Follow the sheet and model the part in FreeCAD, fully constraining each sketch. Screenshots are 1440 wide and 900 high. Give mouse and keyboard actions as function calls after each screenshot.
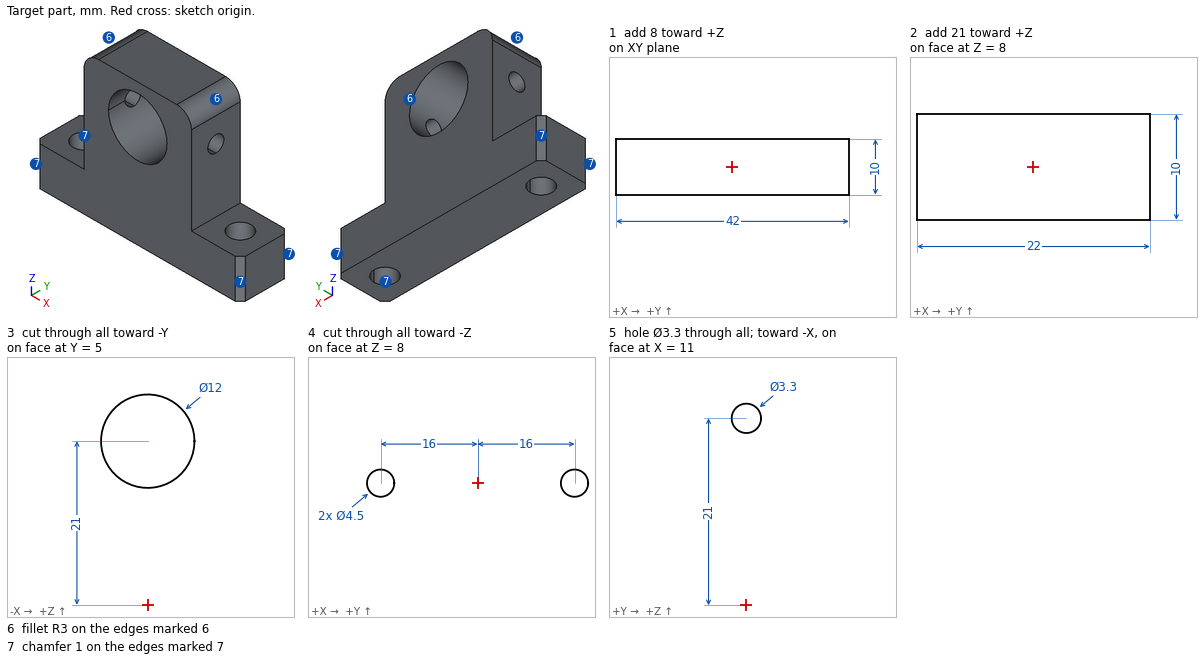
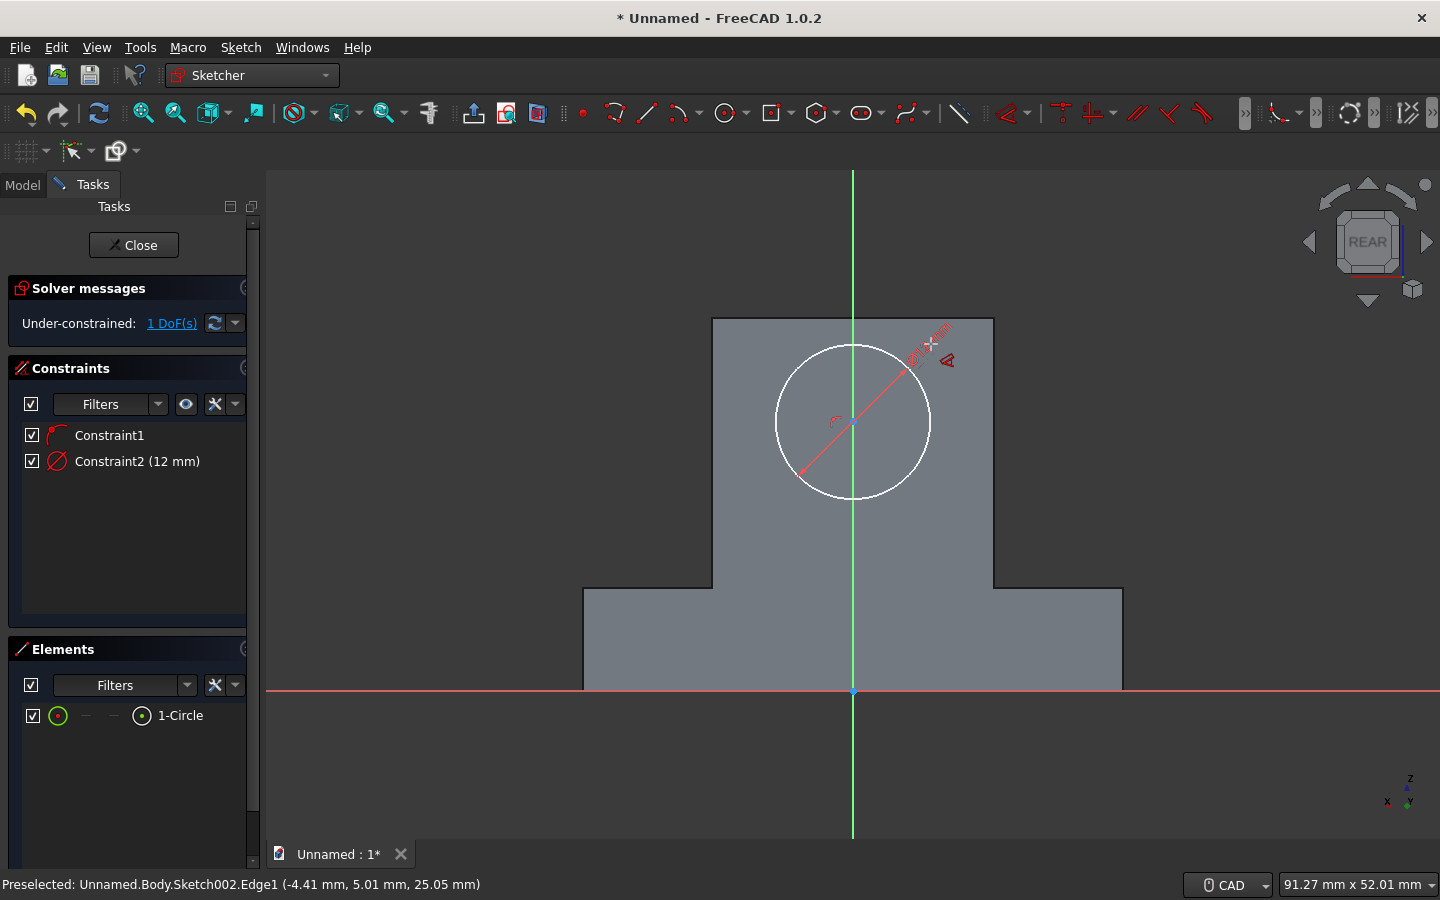
click(853, 422)
click(887, 557)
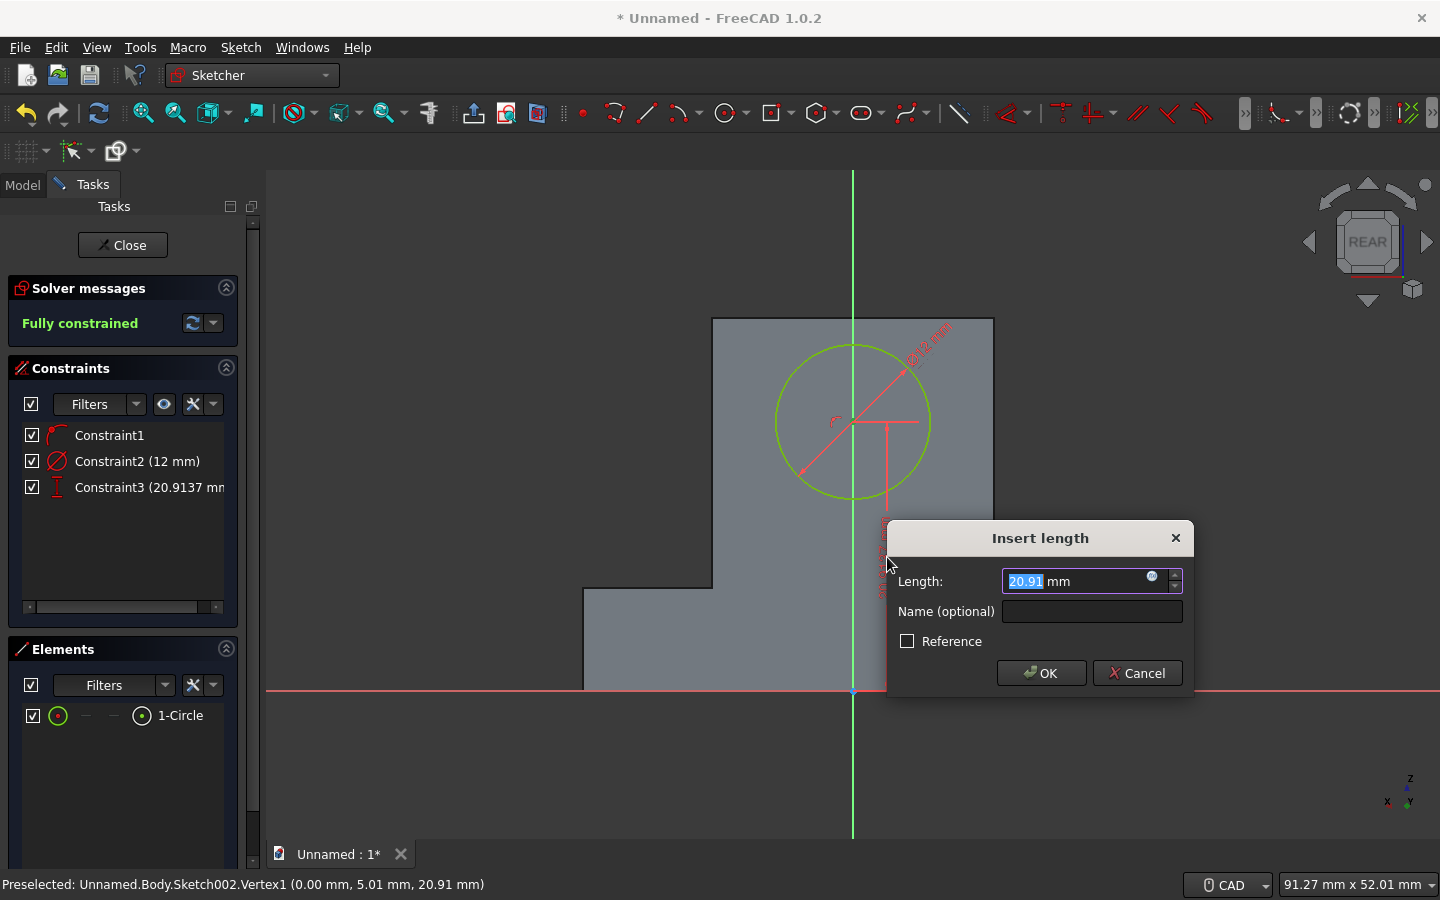
text(21)
key(Return)
key(Escape)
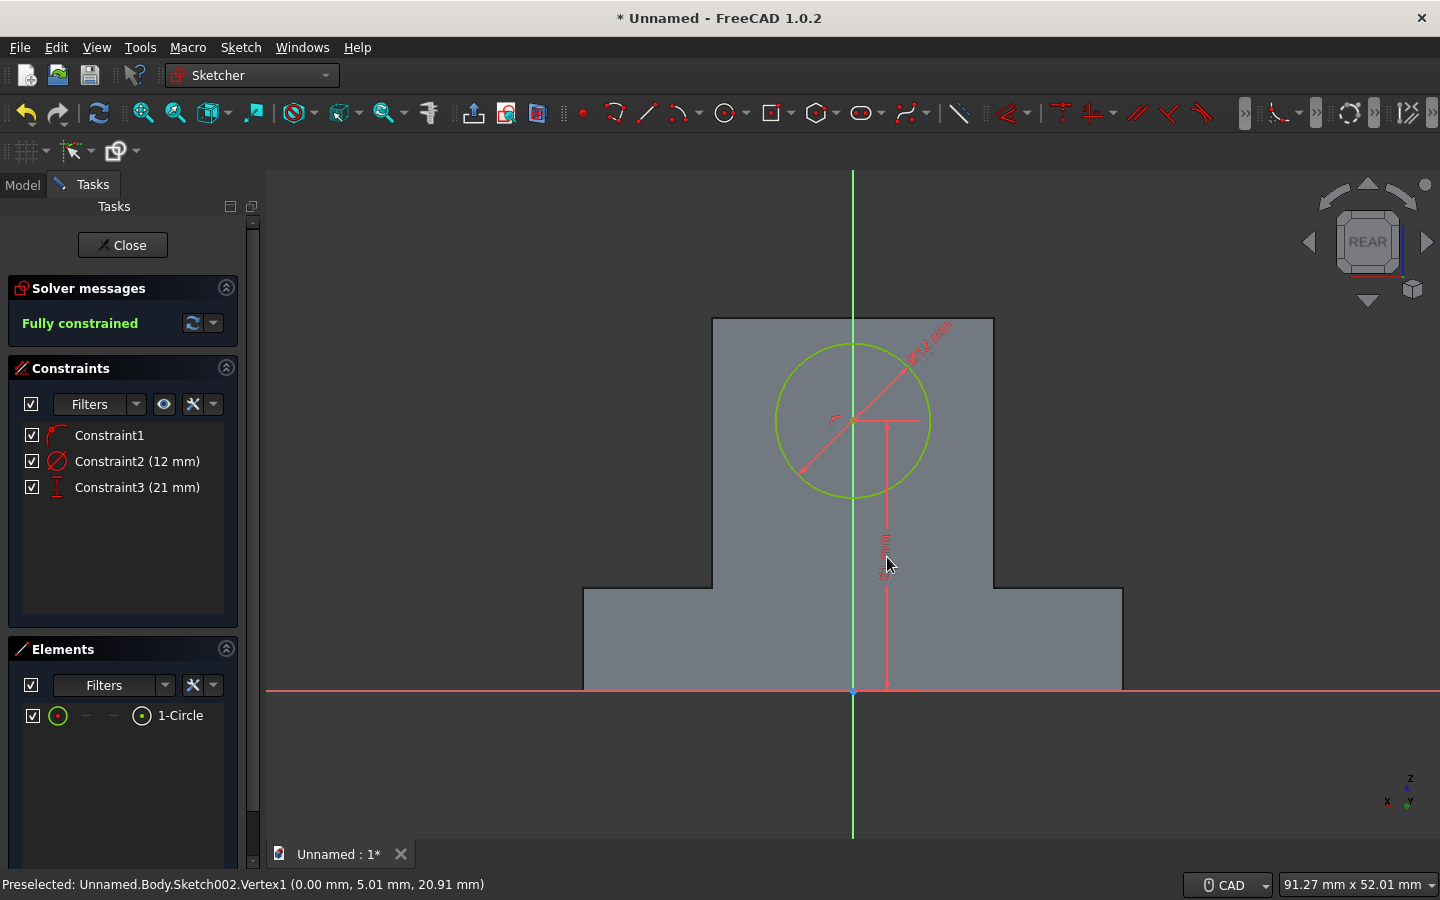
click(123, 245)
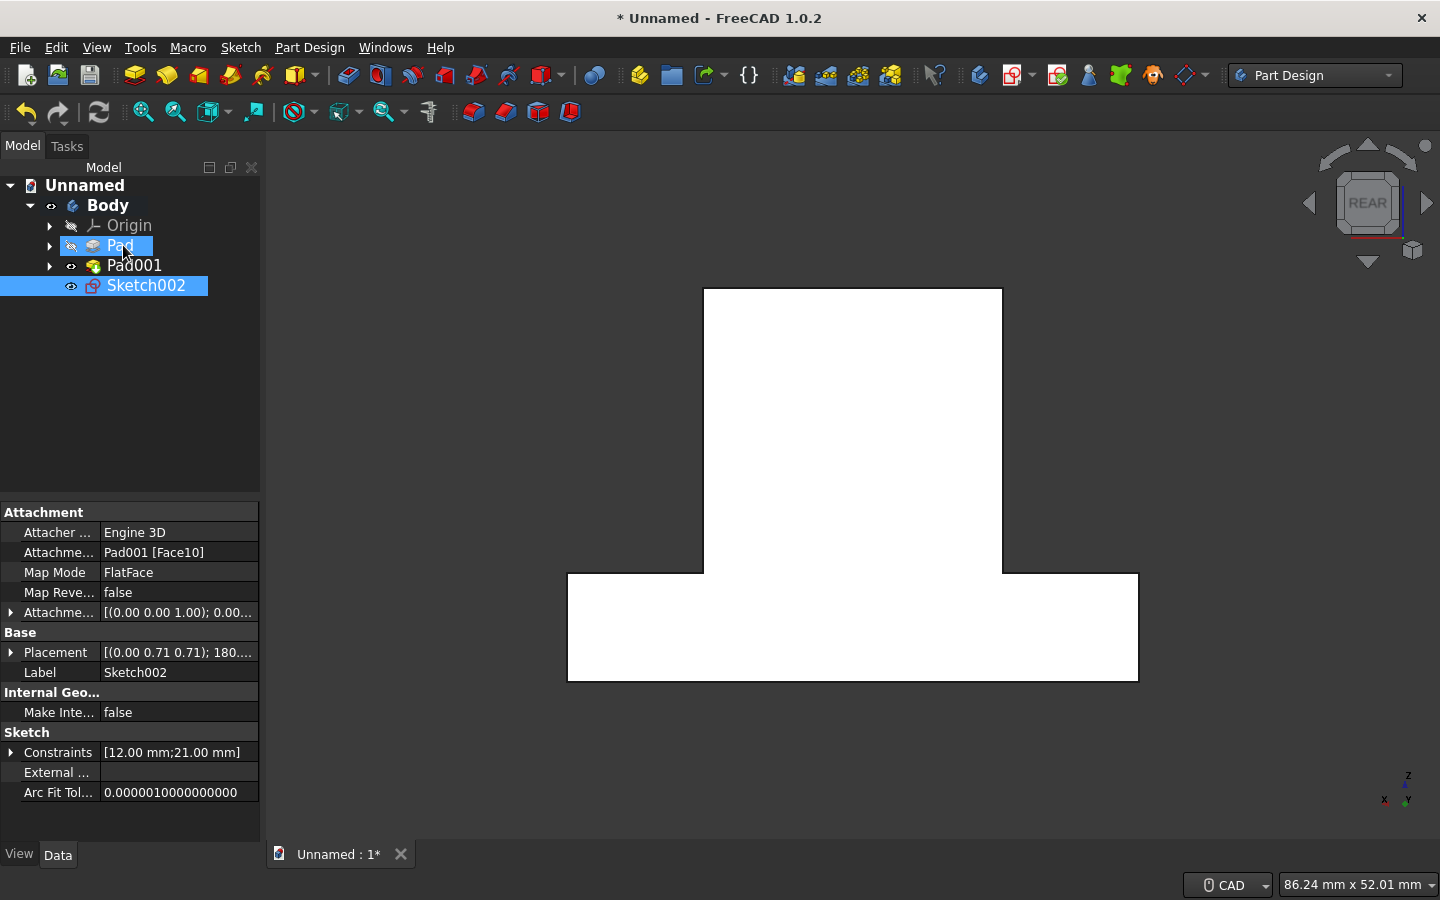
click(350, 76)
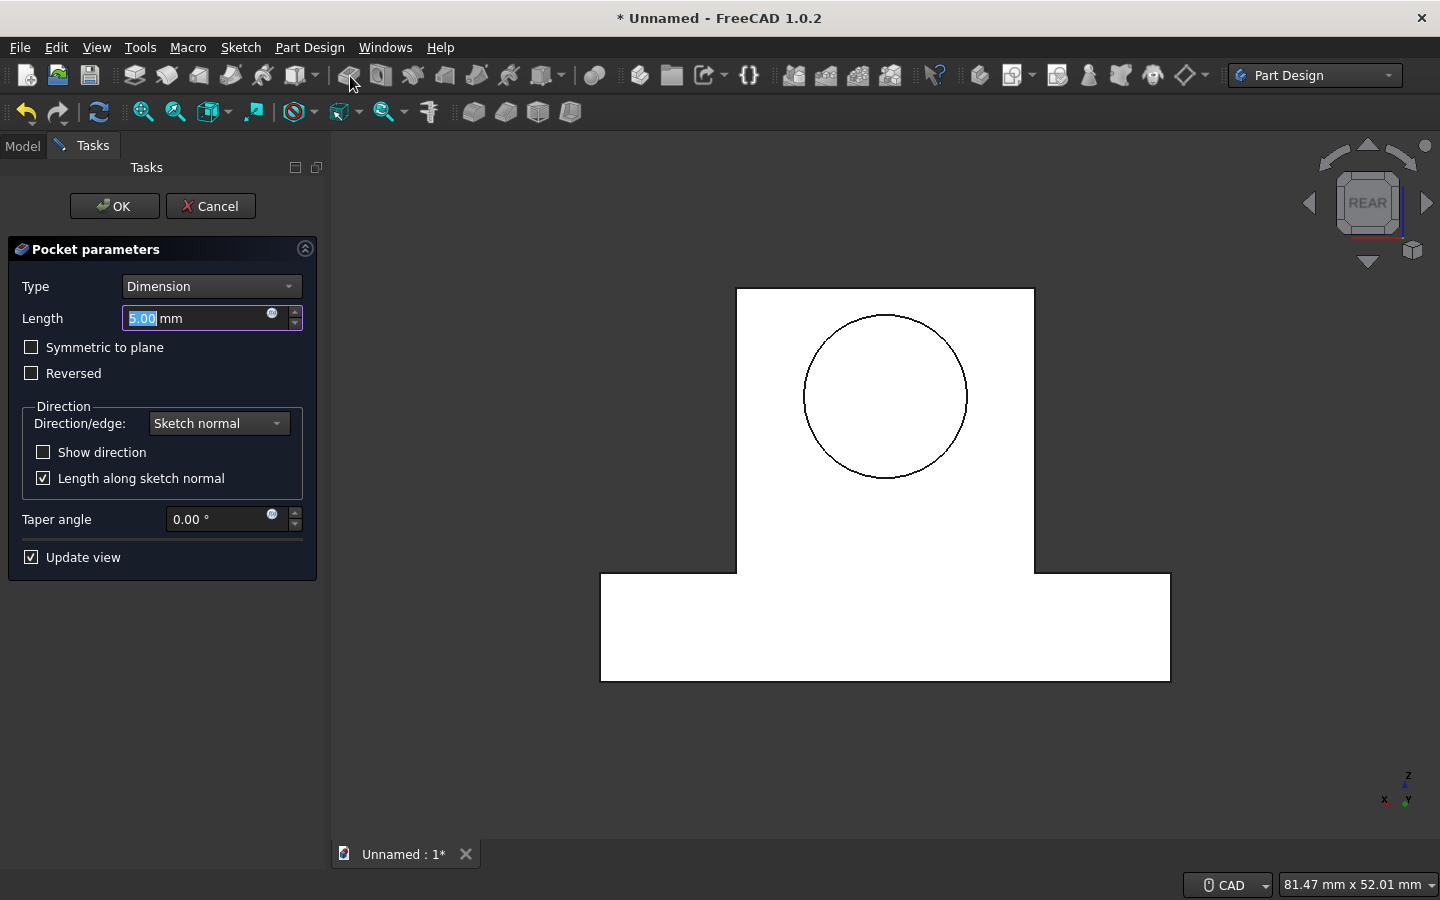
click(212, 286)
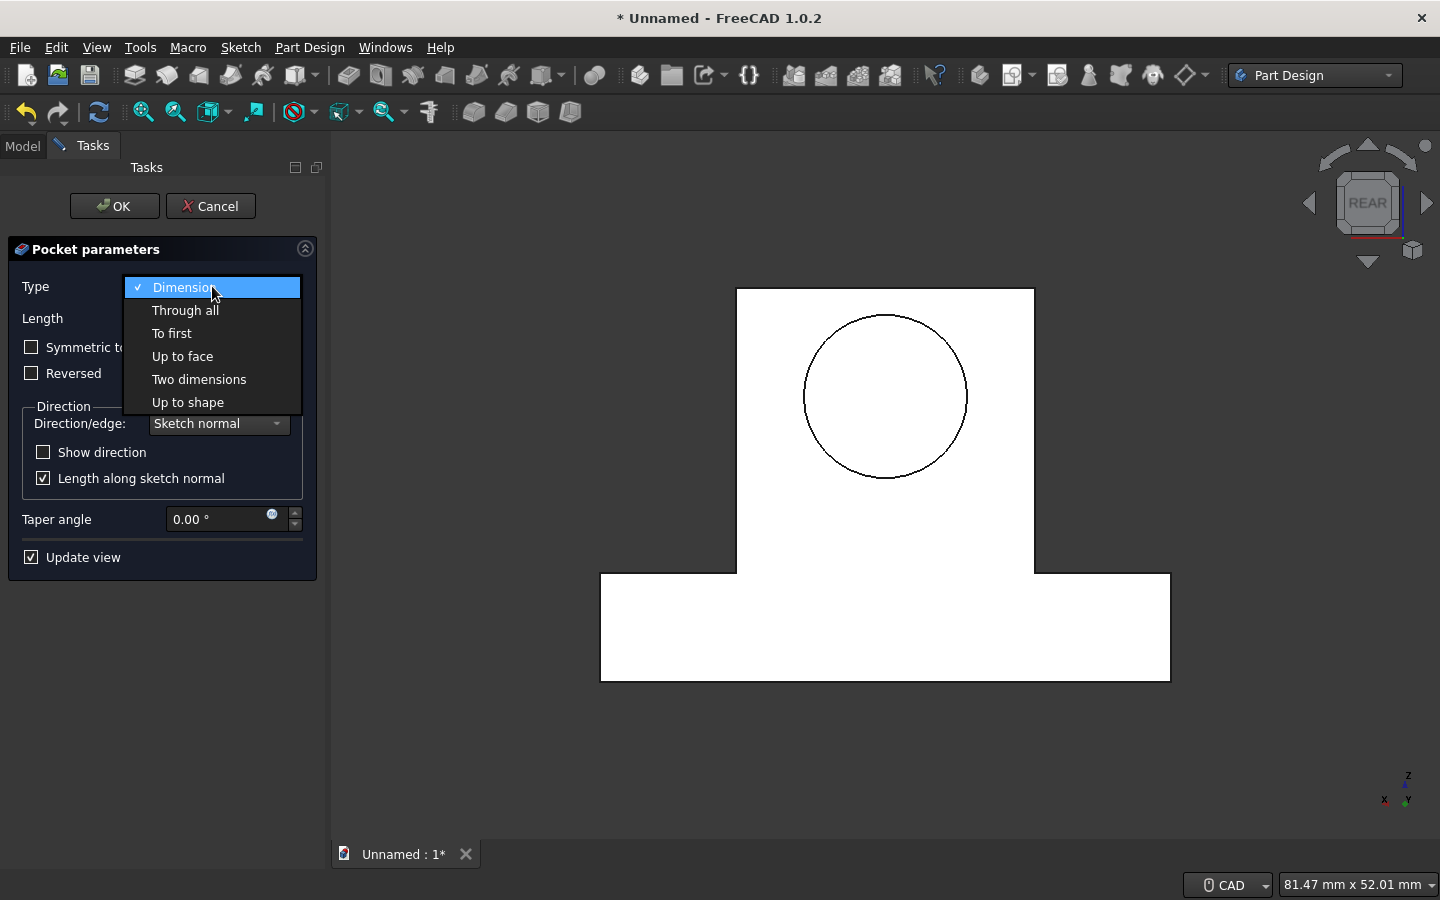
click(212, 310)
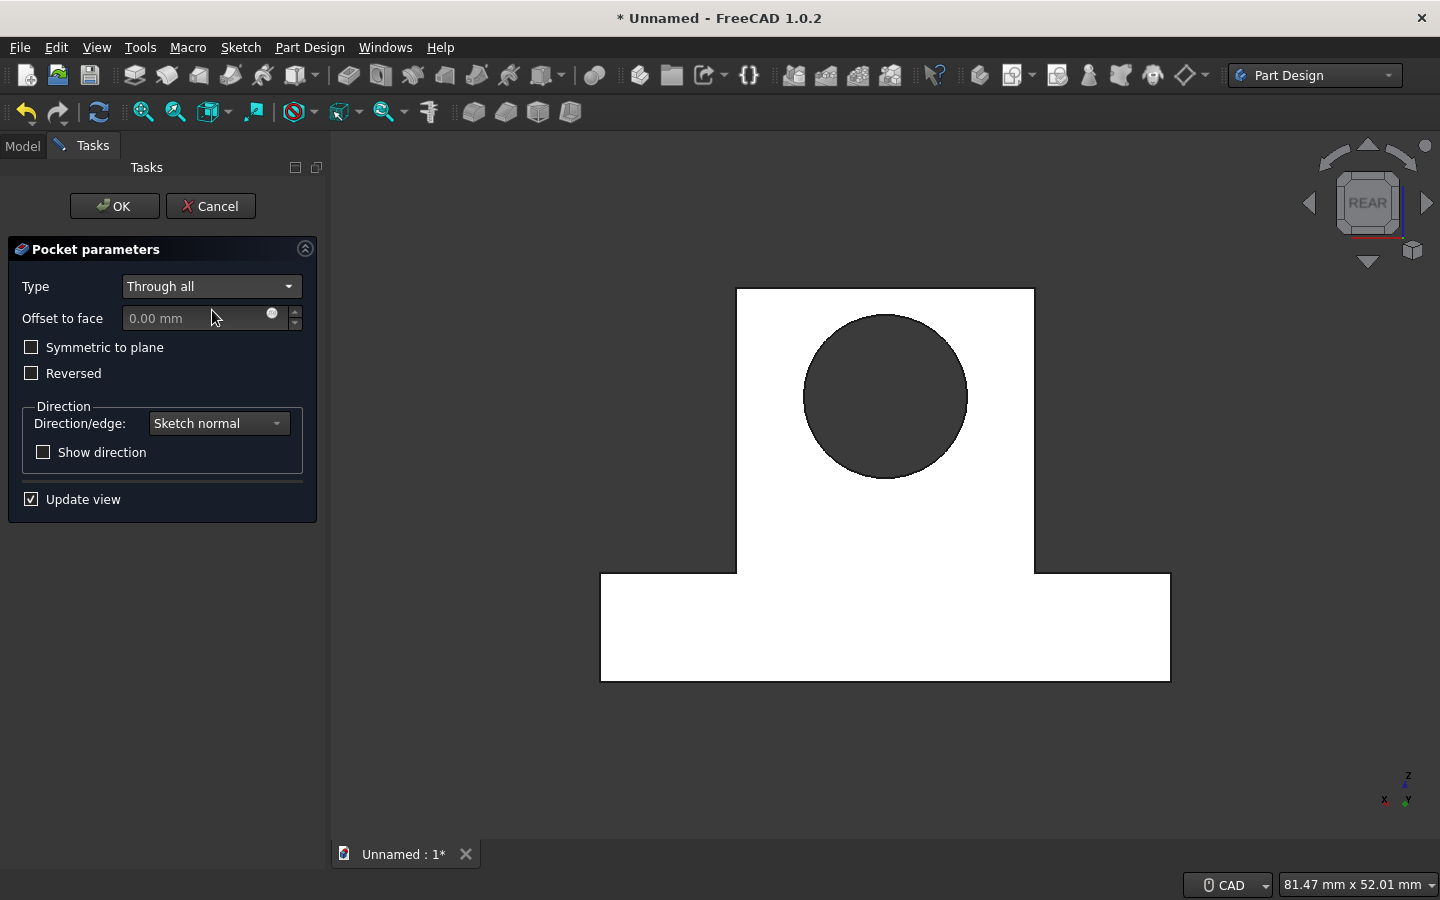
click(115, 206)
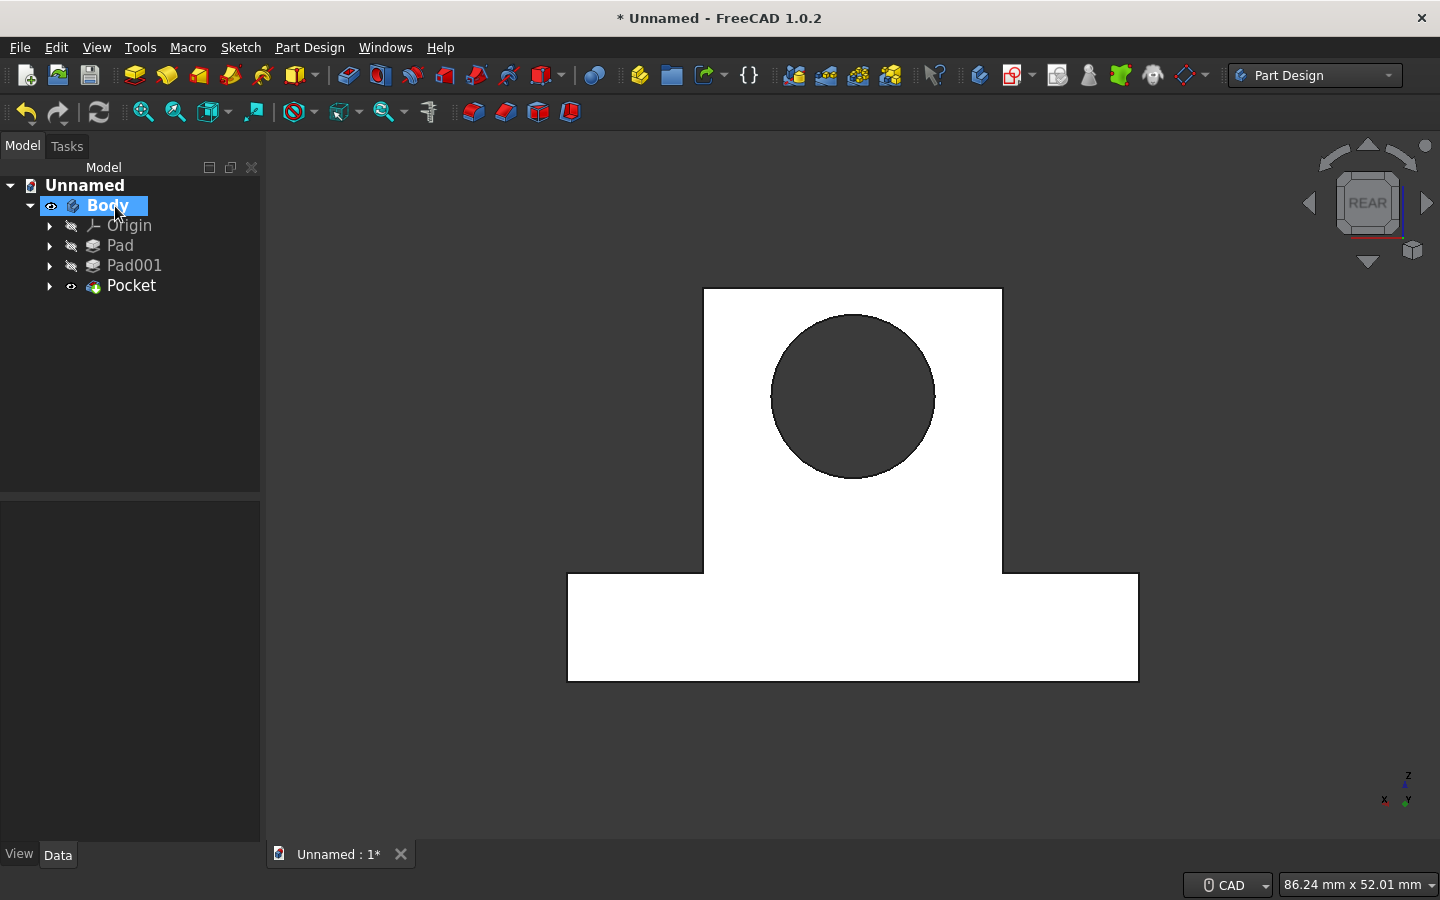
key(0)